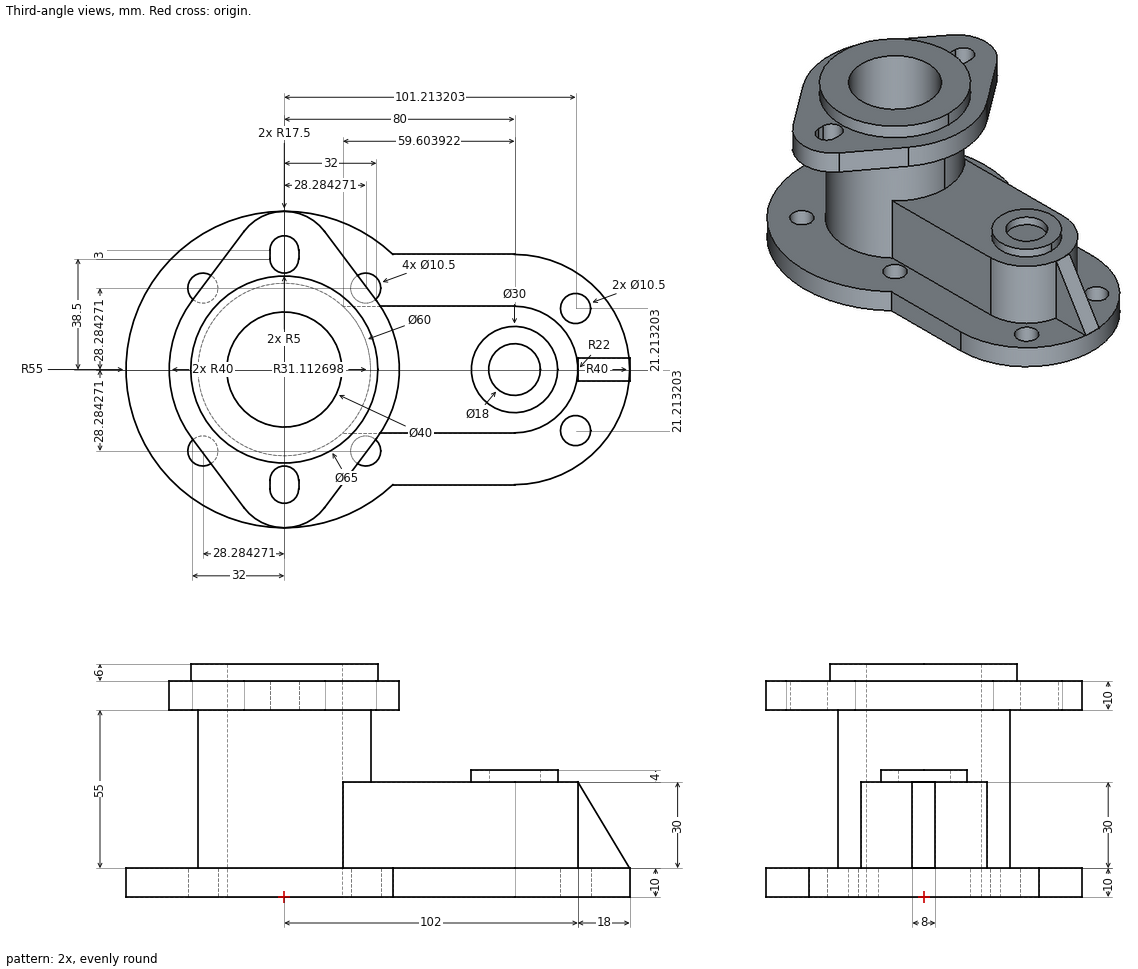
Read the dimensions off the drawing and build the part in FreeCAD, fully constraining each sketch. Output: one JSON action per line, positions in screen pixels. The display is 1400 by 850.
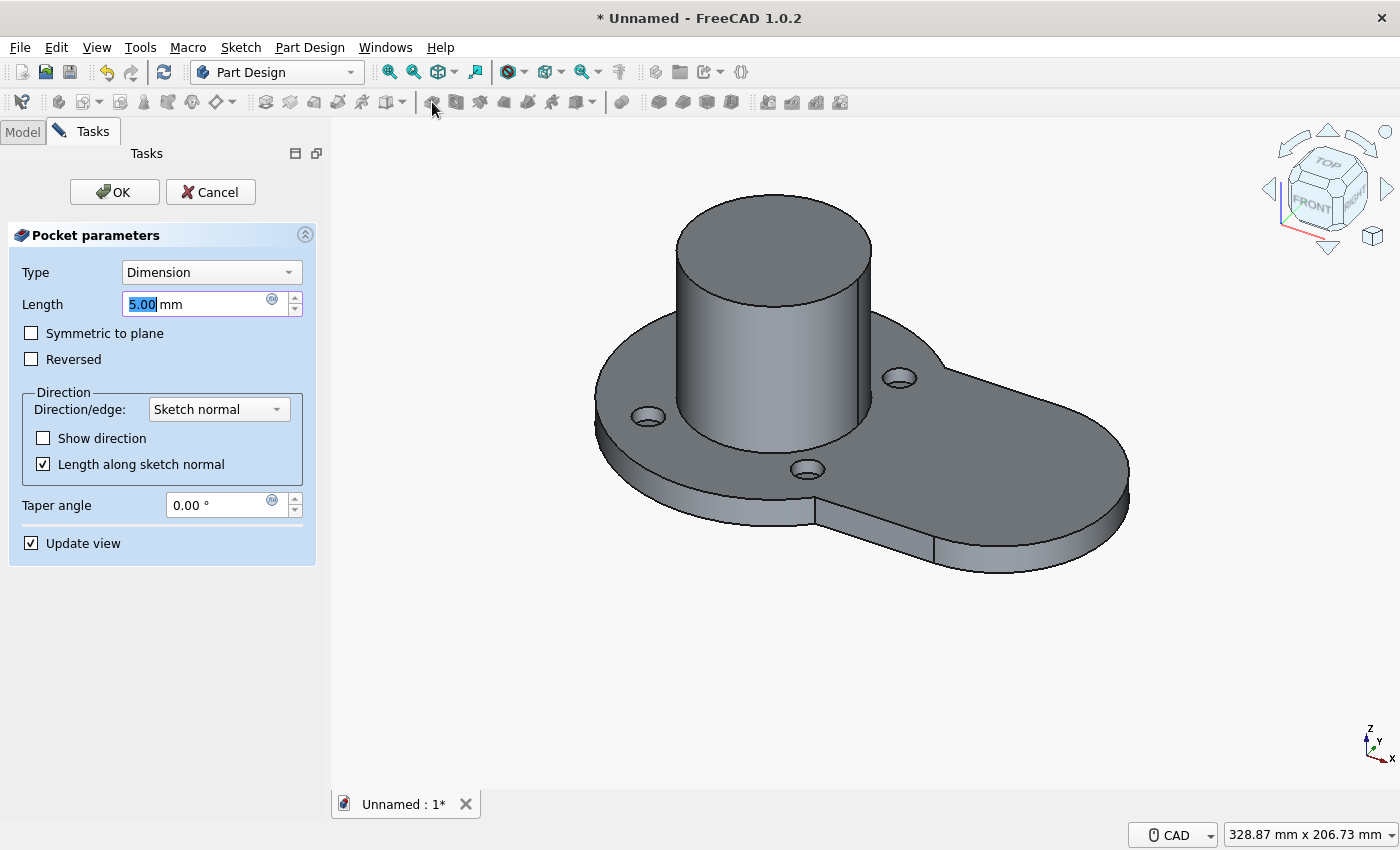
{"action": "left_click", "coordinate": [212, 272]}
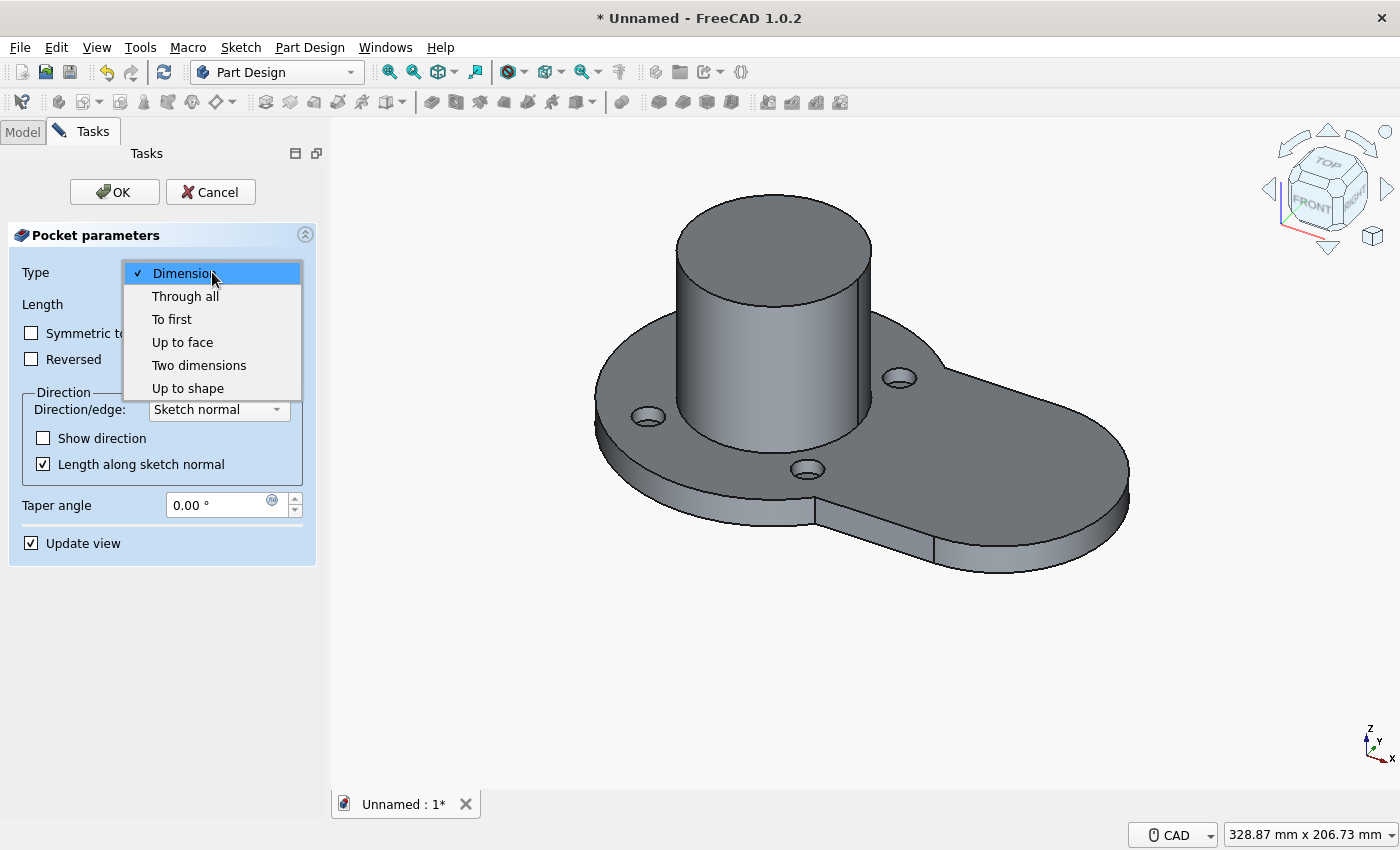
{"action": "left_click", "coordinate": [212, 296]}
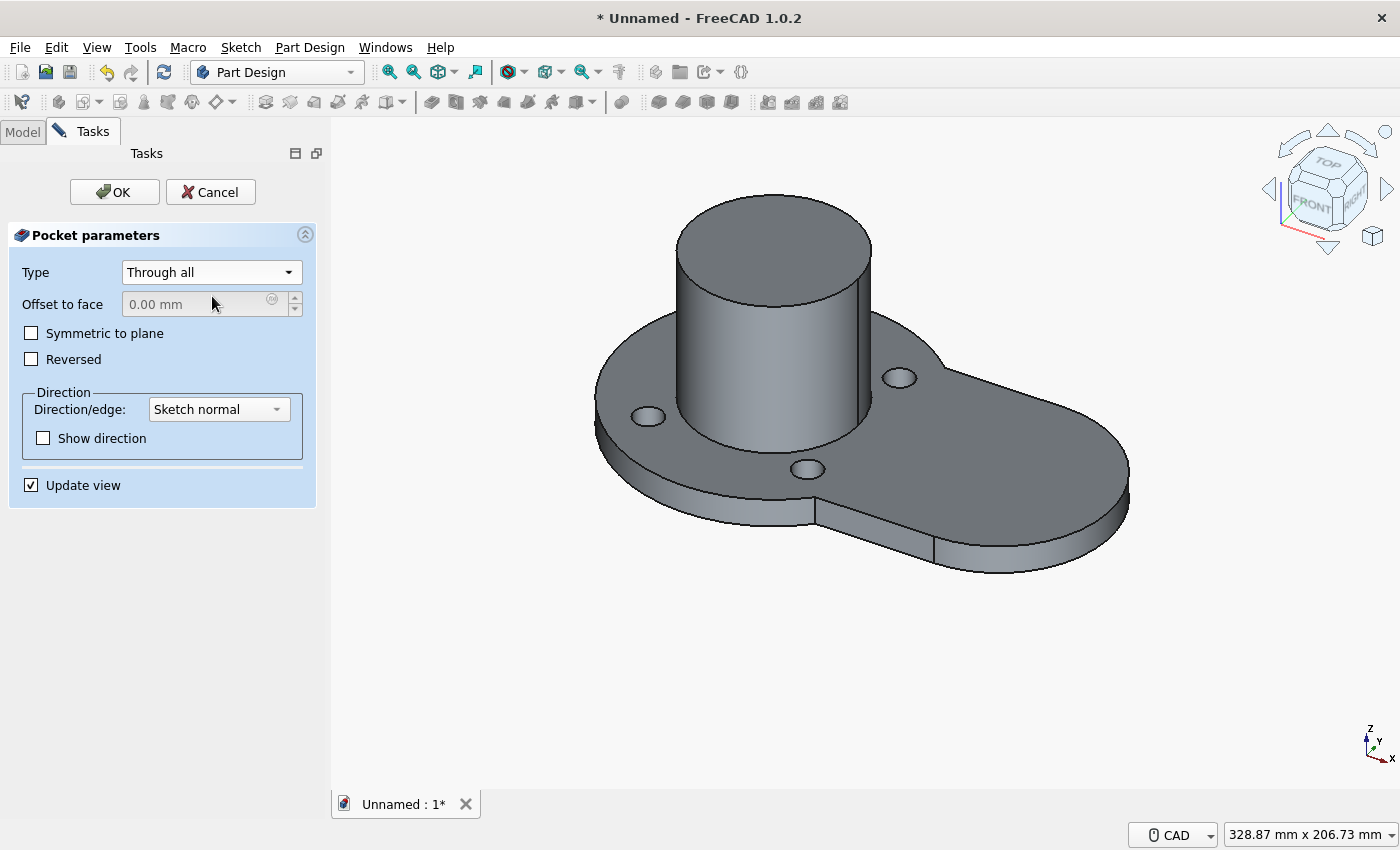
{"action": "left_click", "coordinate": [115, 192]}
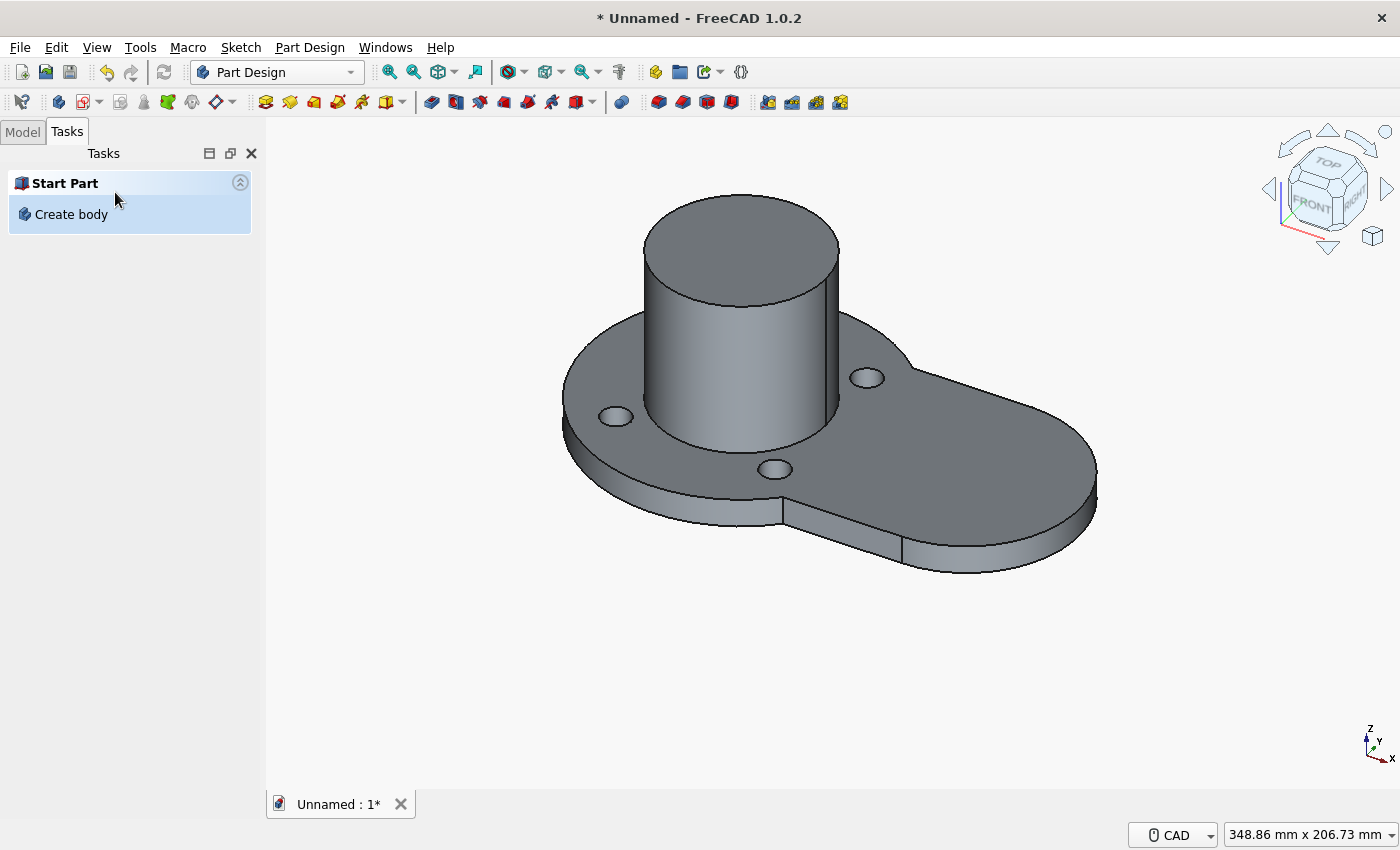
{"action": "left_click", "coordinate": [390, 72]}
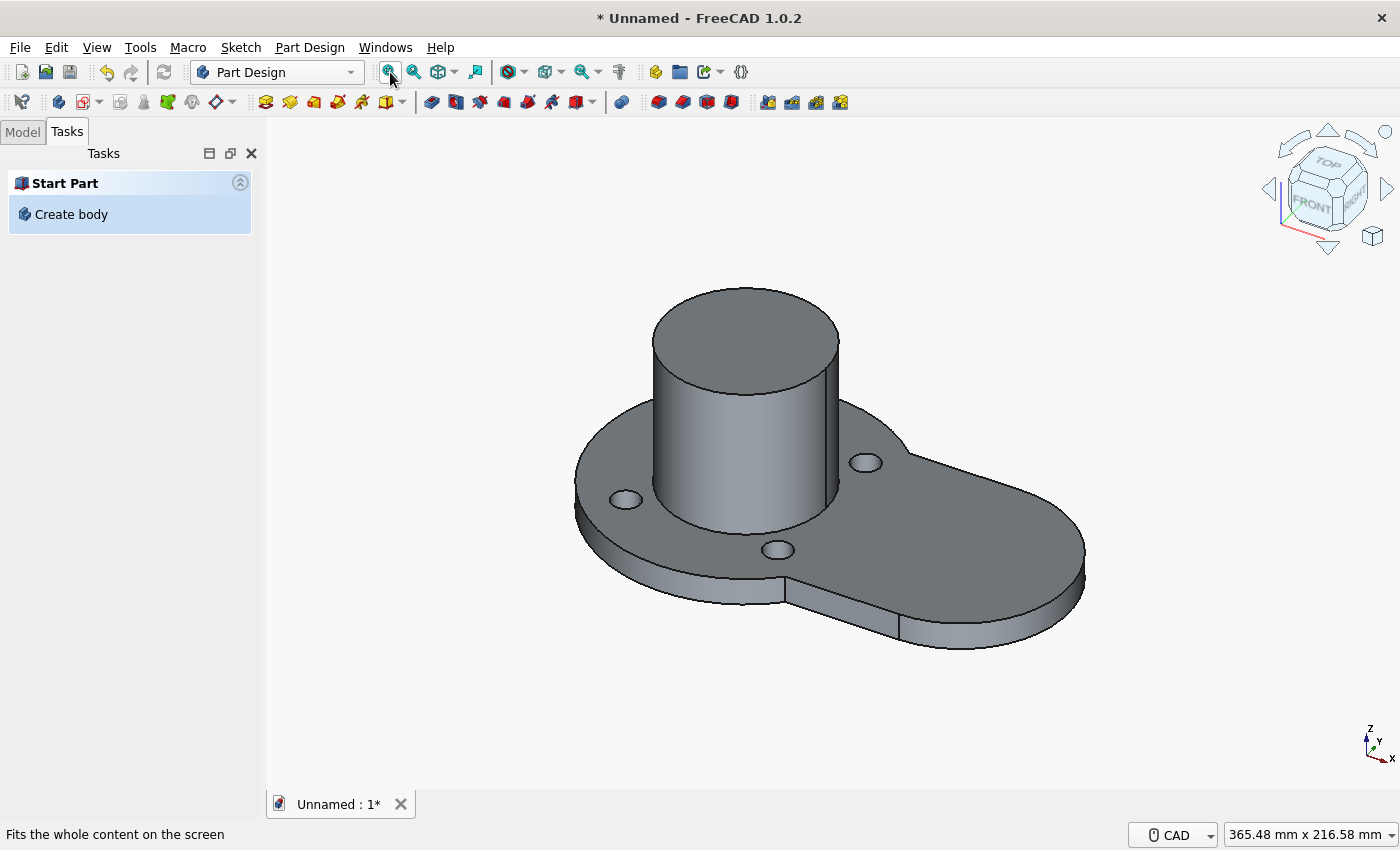
{"action": "left_click", "coordinate": [968, 554]}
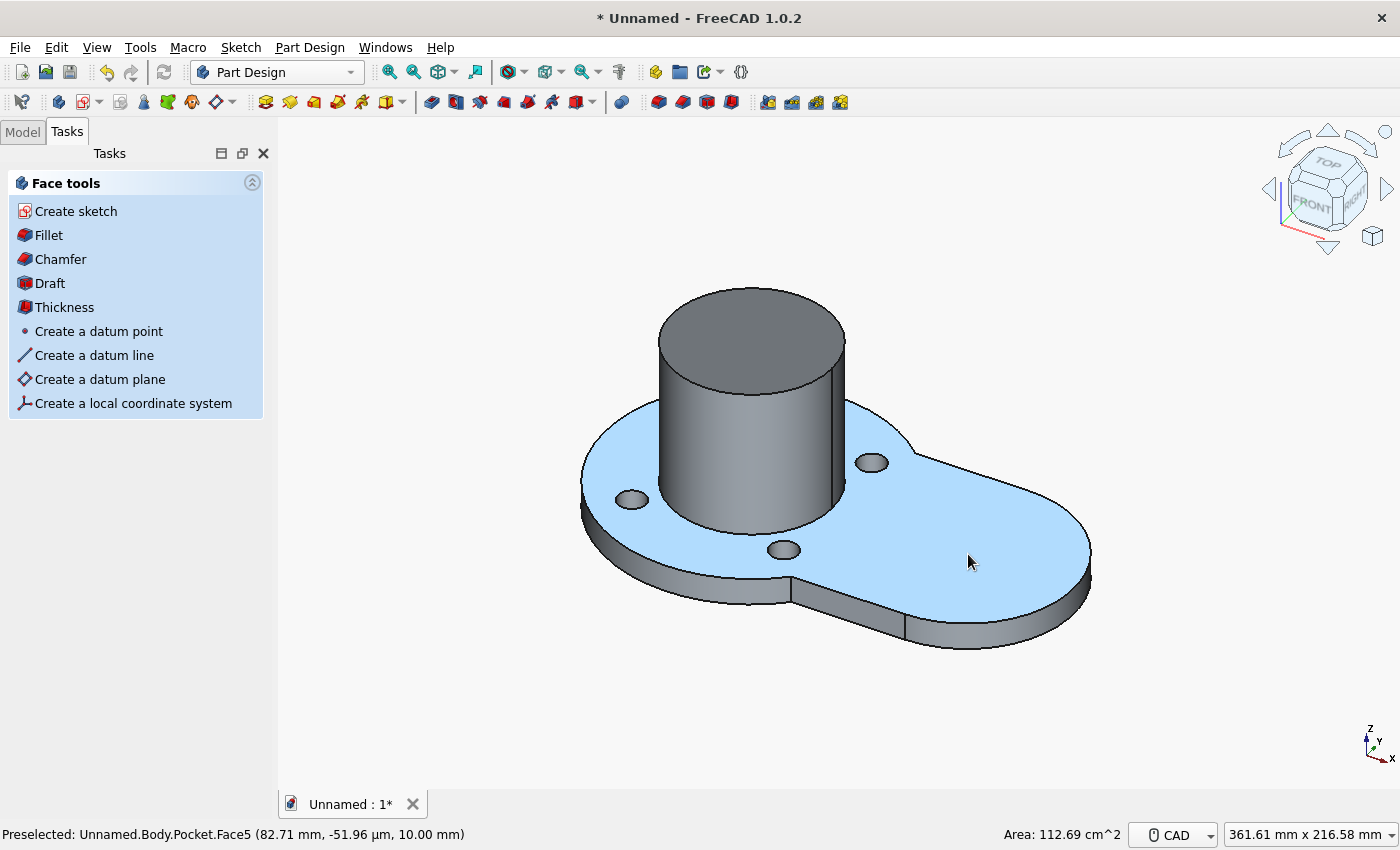
{"action": "left_click", "coordinate": [84, 102]}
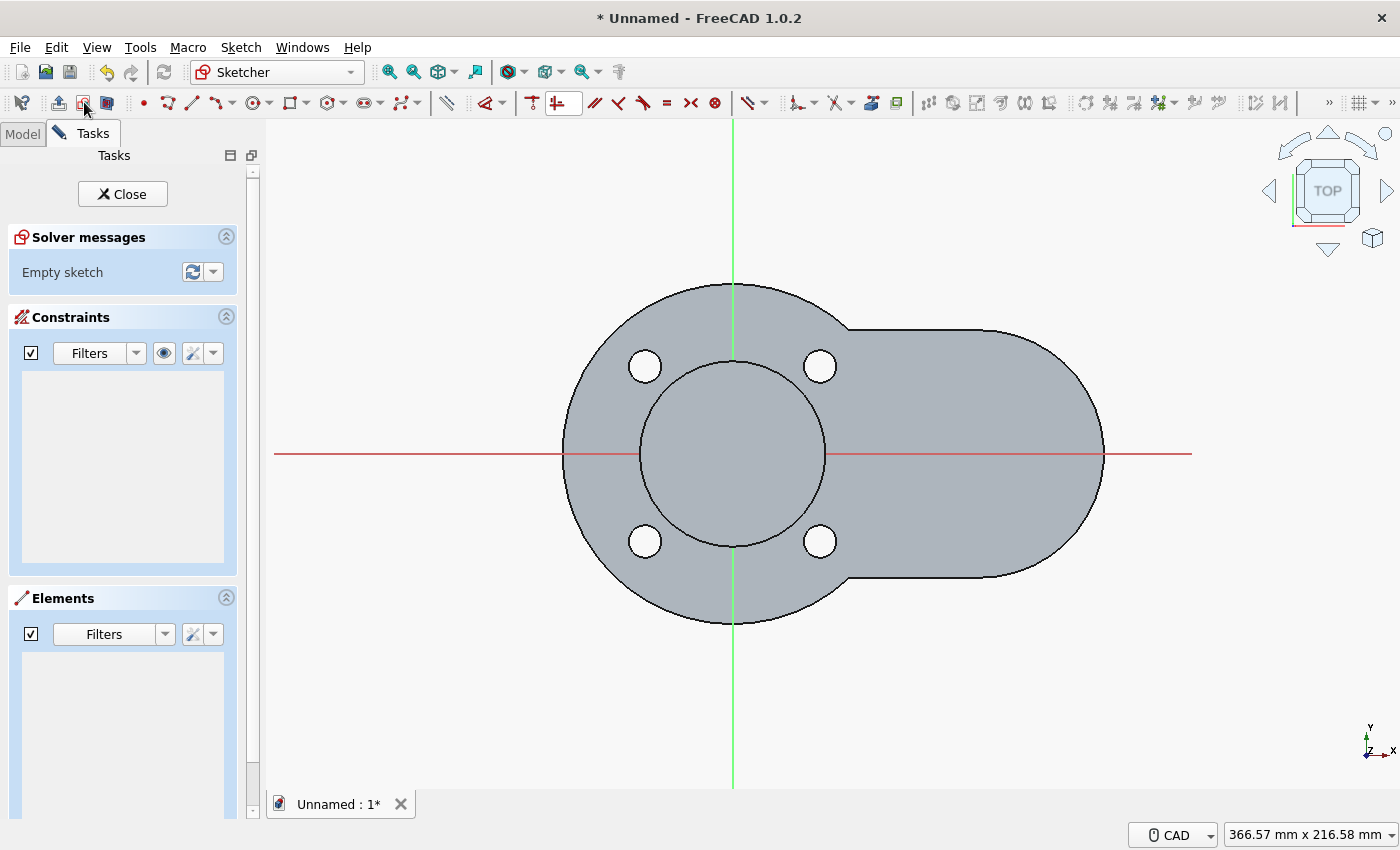
{"action": "scroll", "coordinate": [1006, 454], "scroll_direction": "up", "scroll_amount": 4}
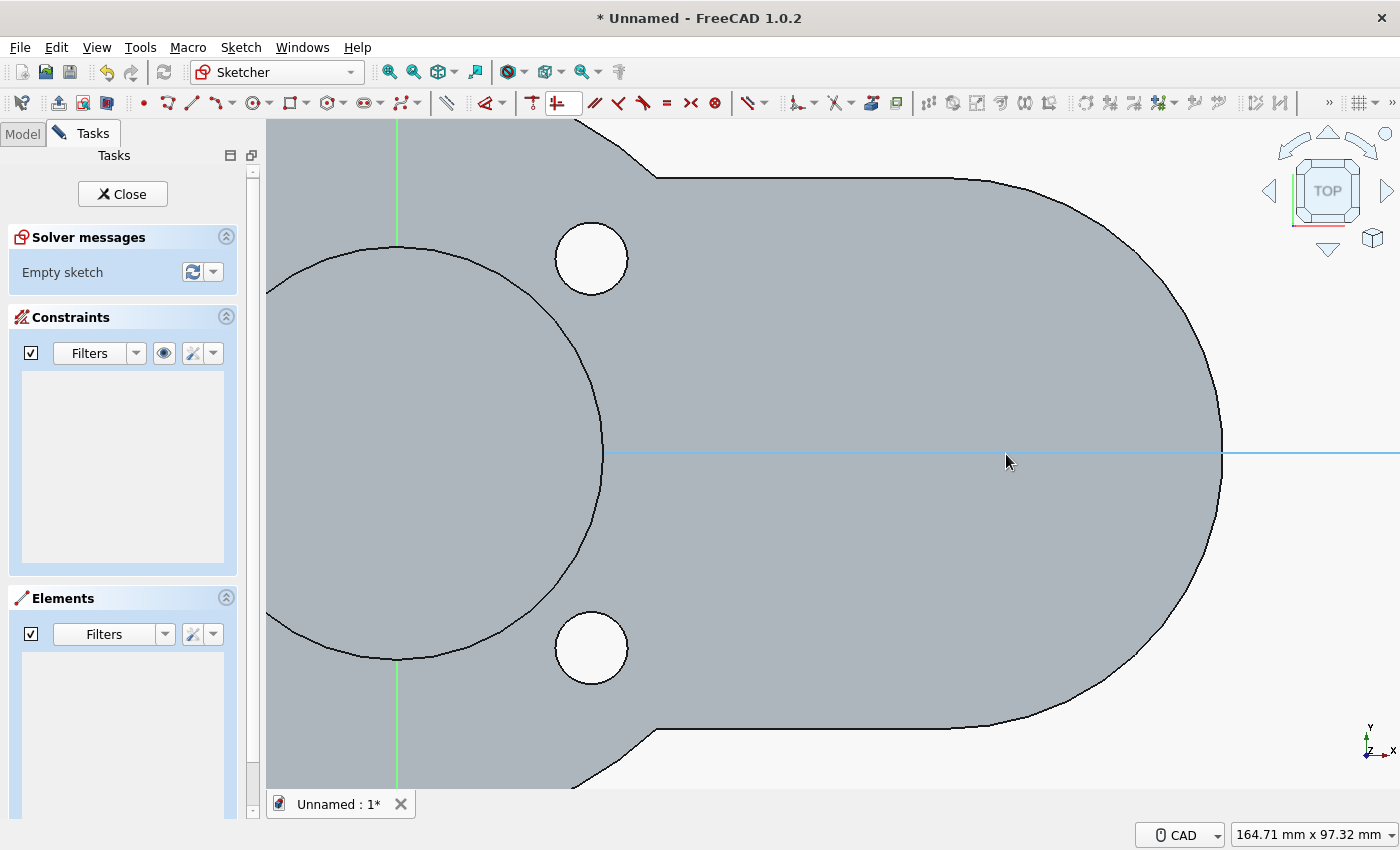
{"action": "left_click", "coordinate": [254, 104]}